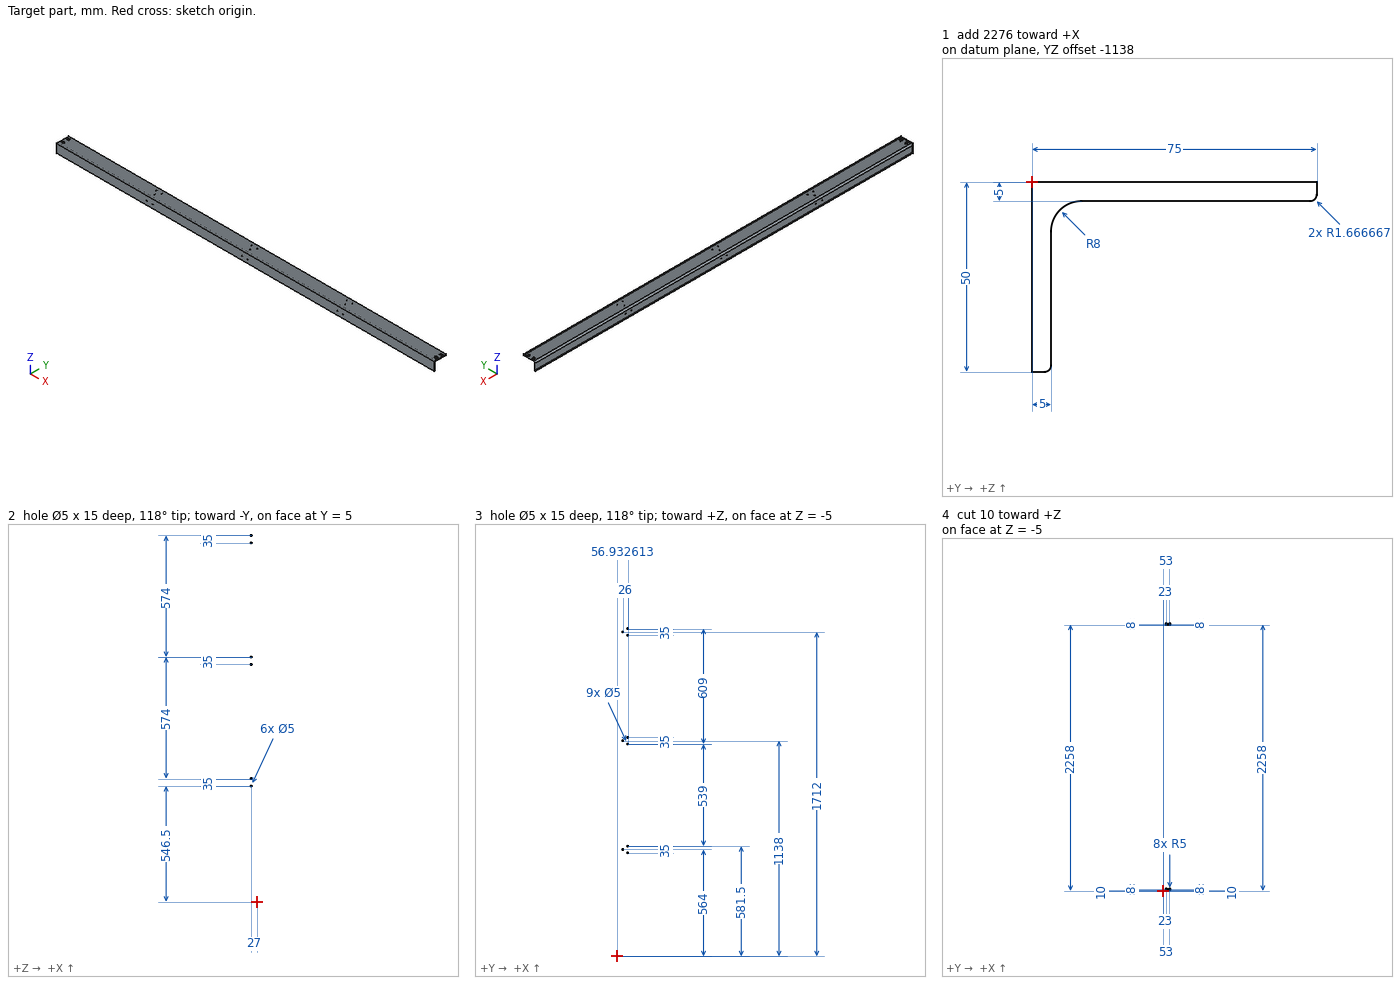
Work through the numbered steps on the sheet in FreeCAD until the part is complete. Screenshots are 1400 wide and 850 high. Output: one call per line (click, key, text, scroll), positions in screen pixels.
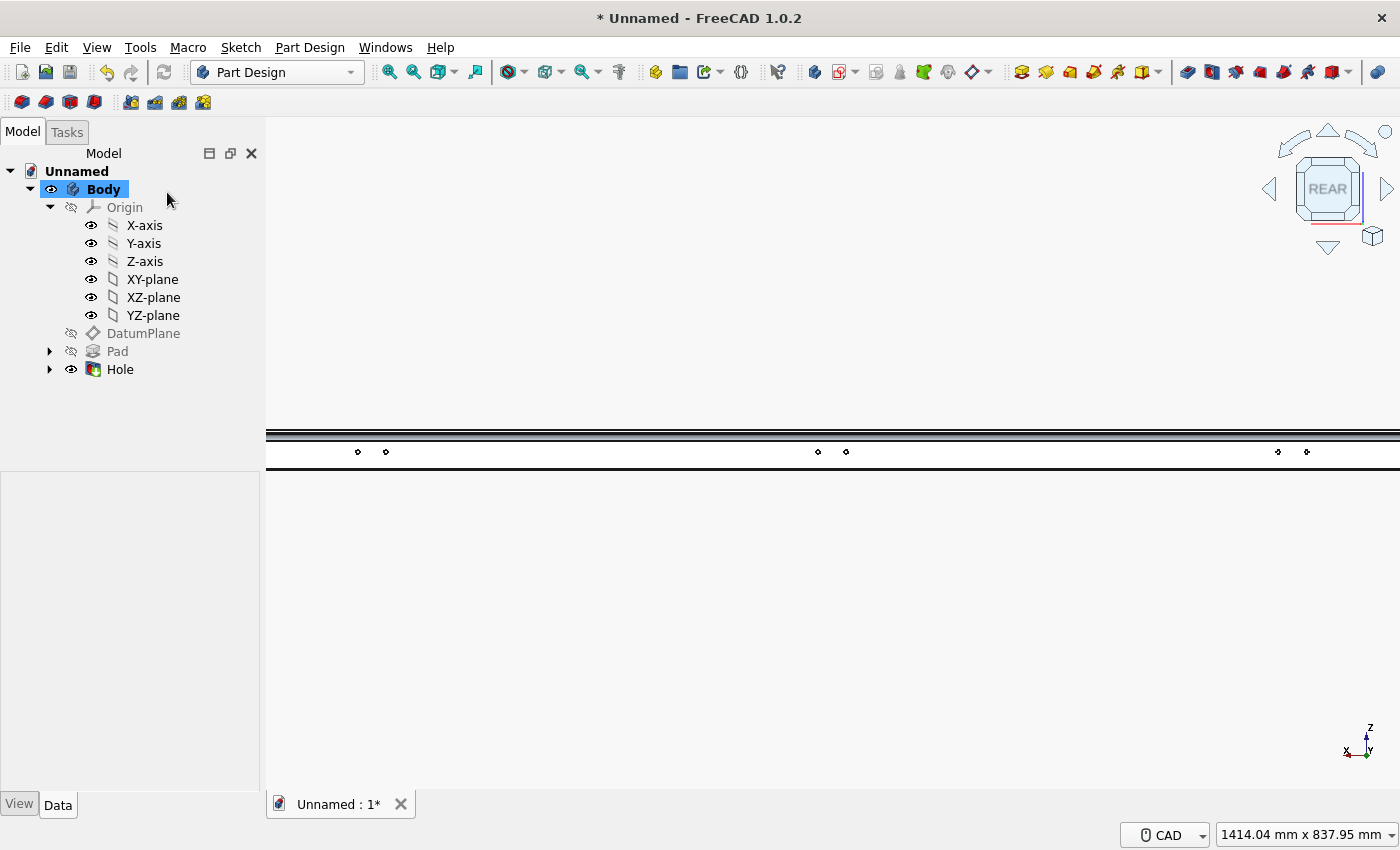
click(390, 72)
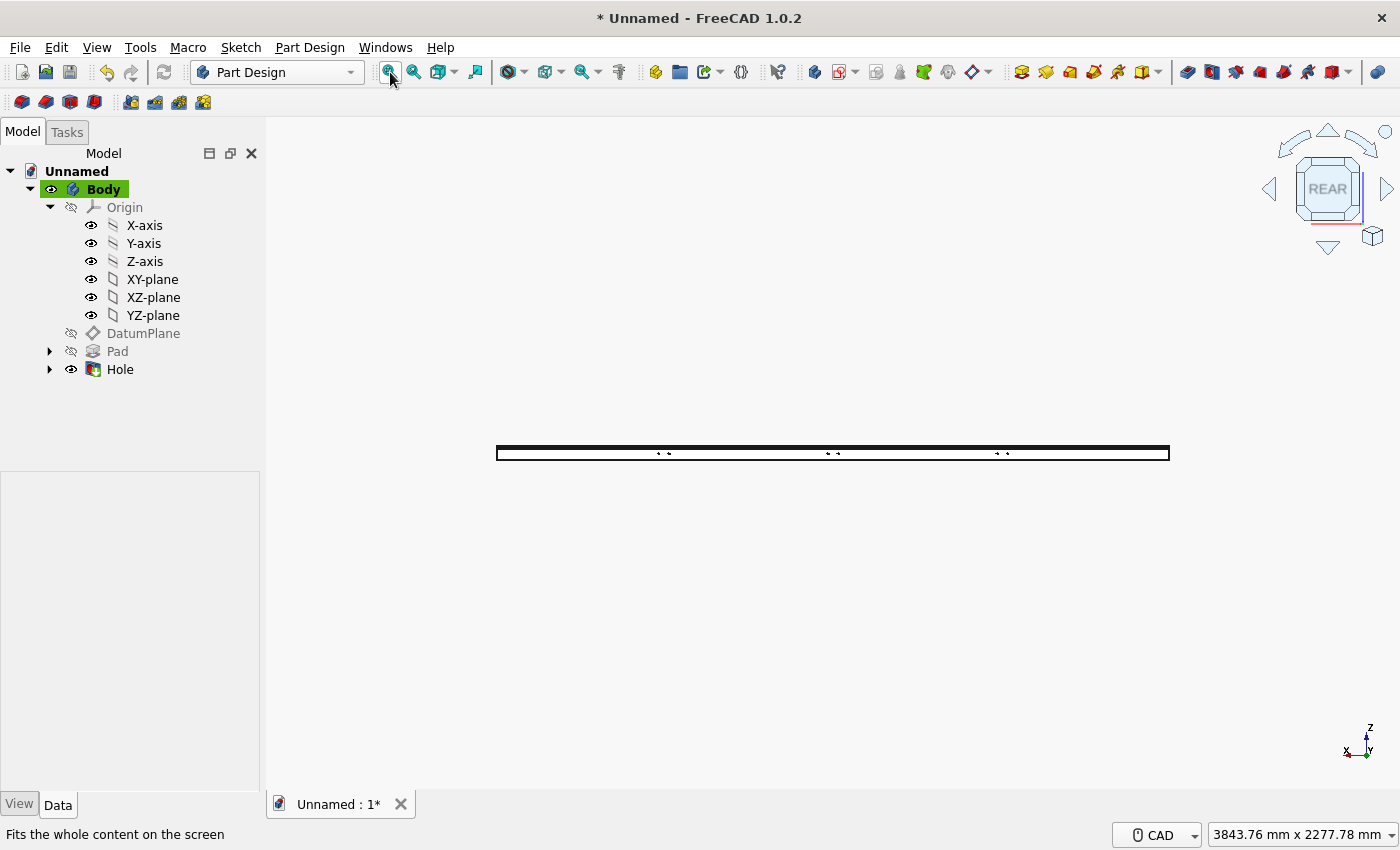
key(5)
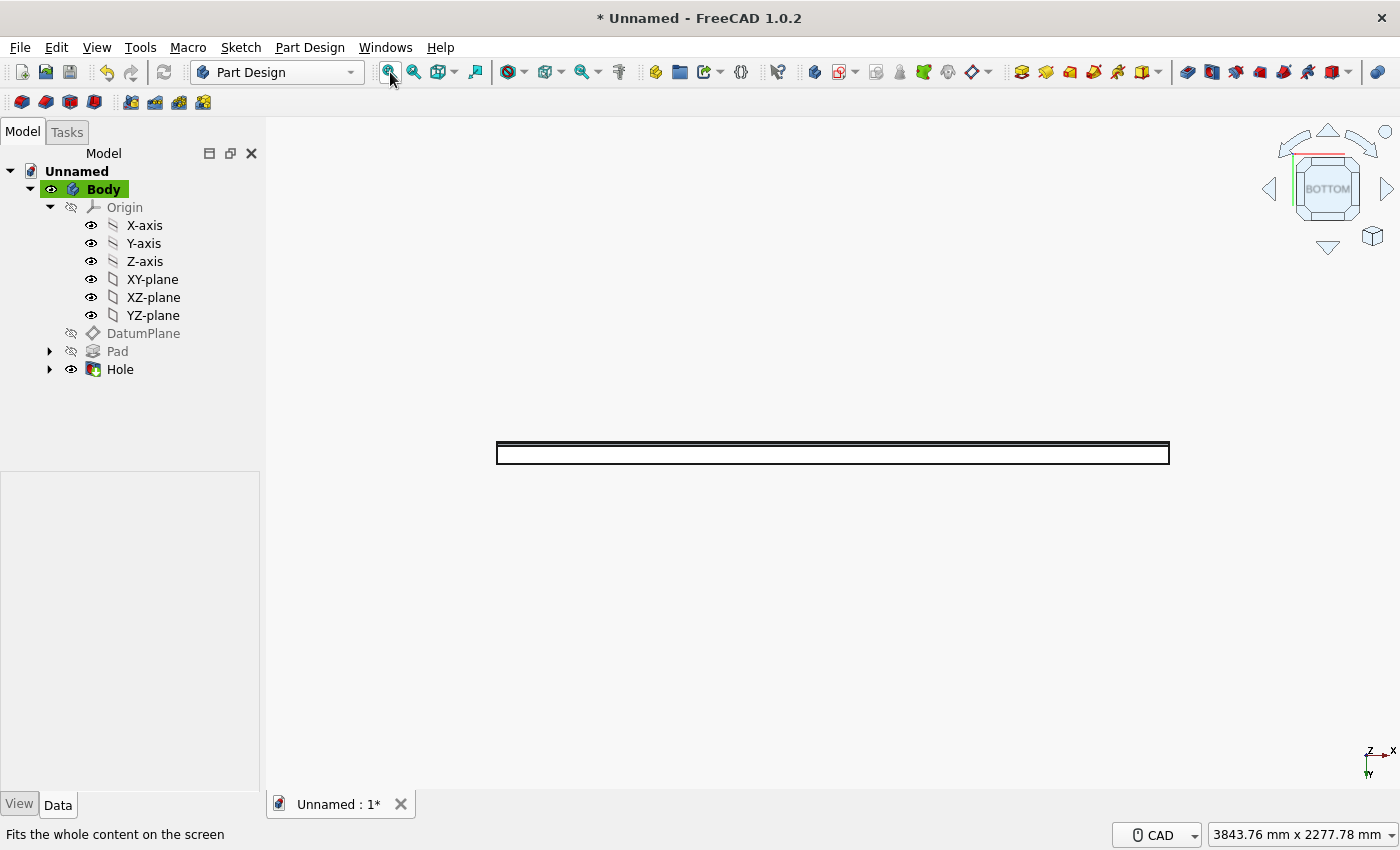
click(833, 454)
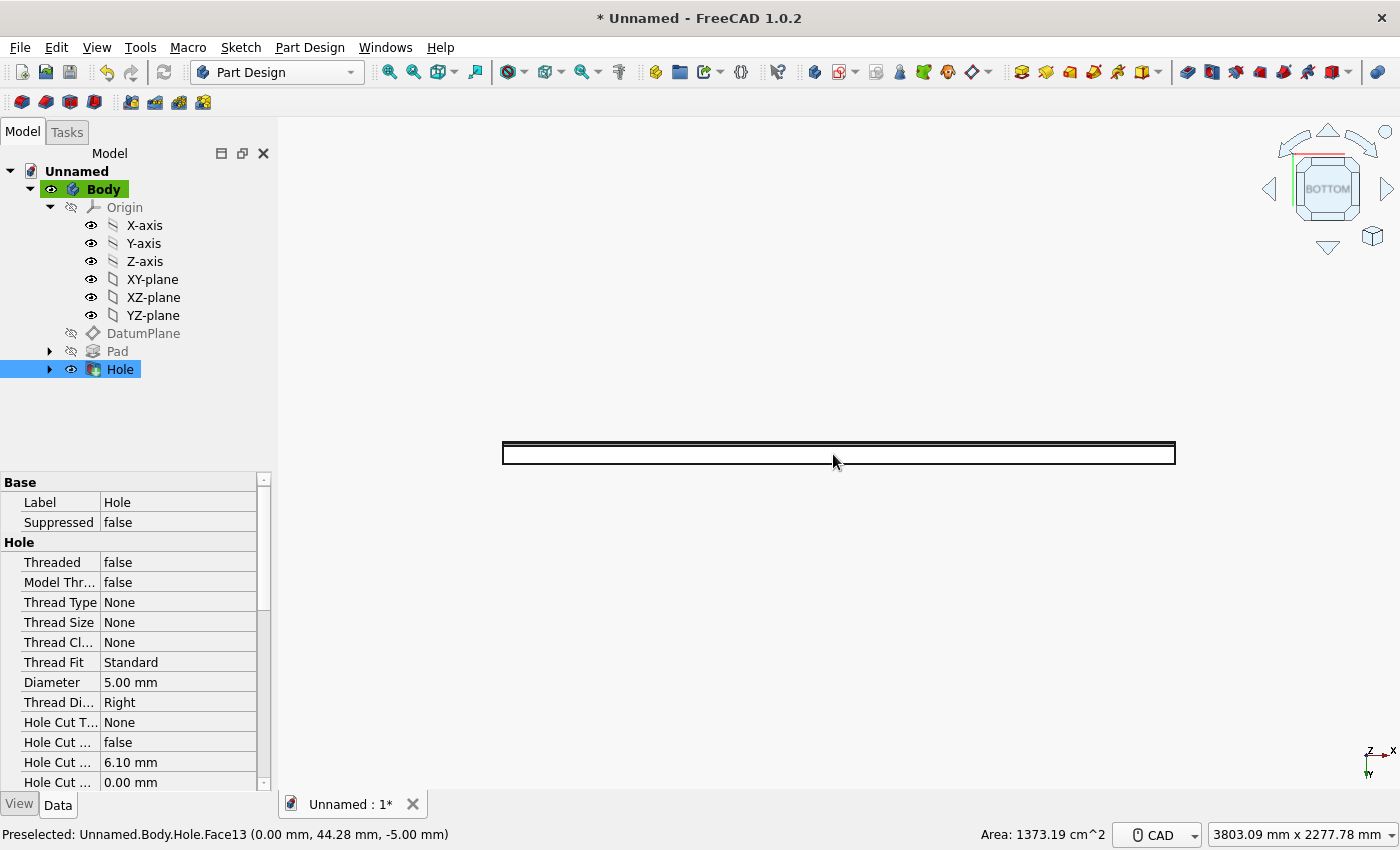
click(840, 72)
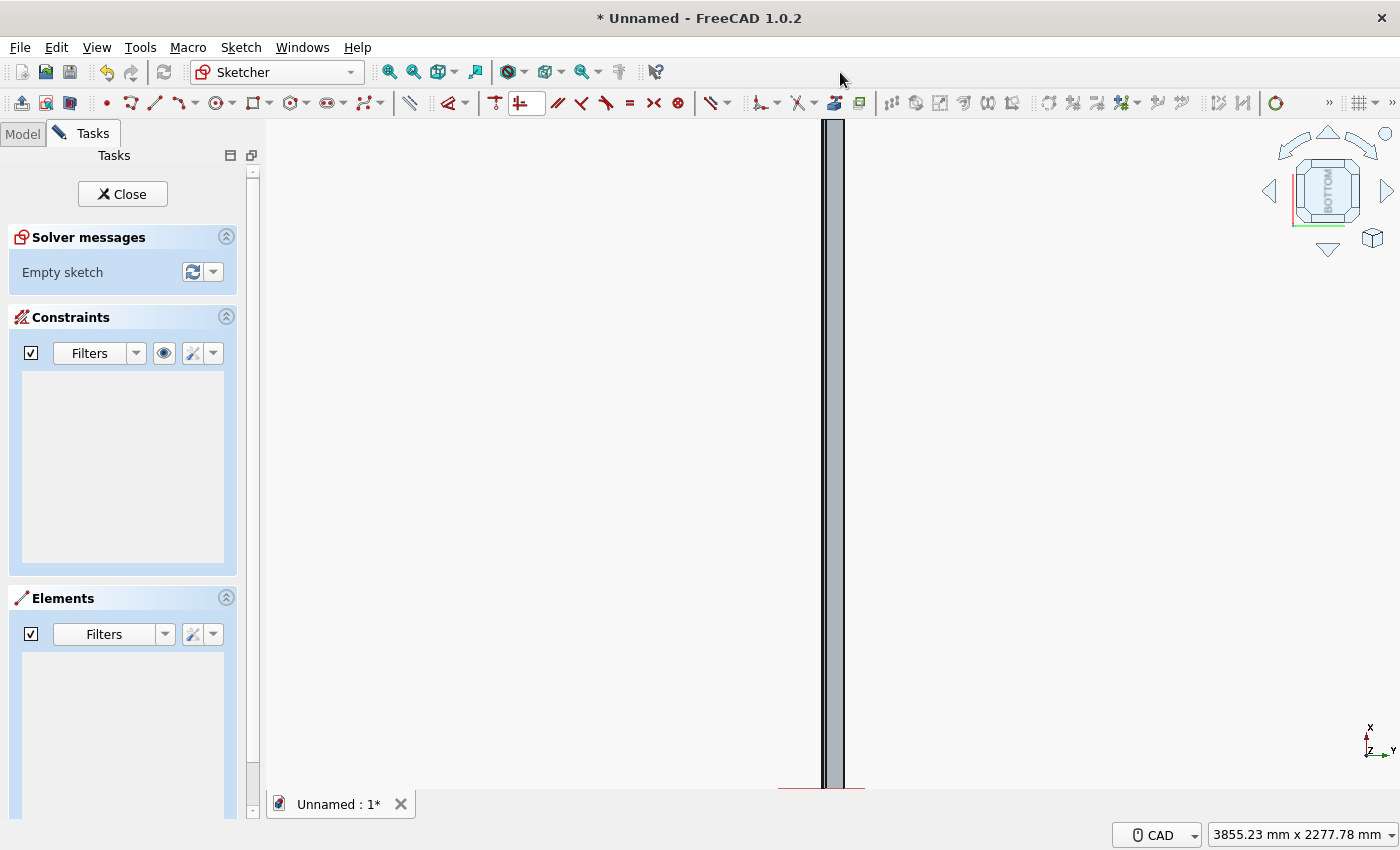
click(70, 104)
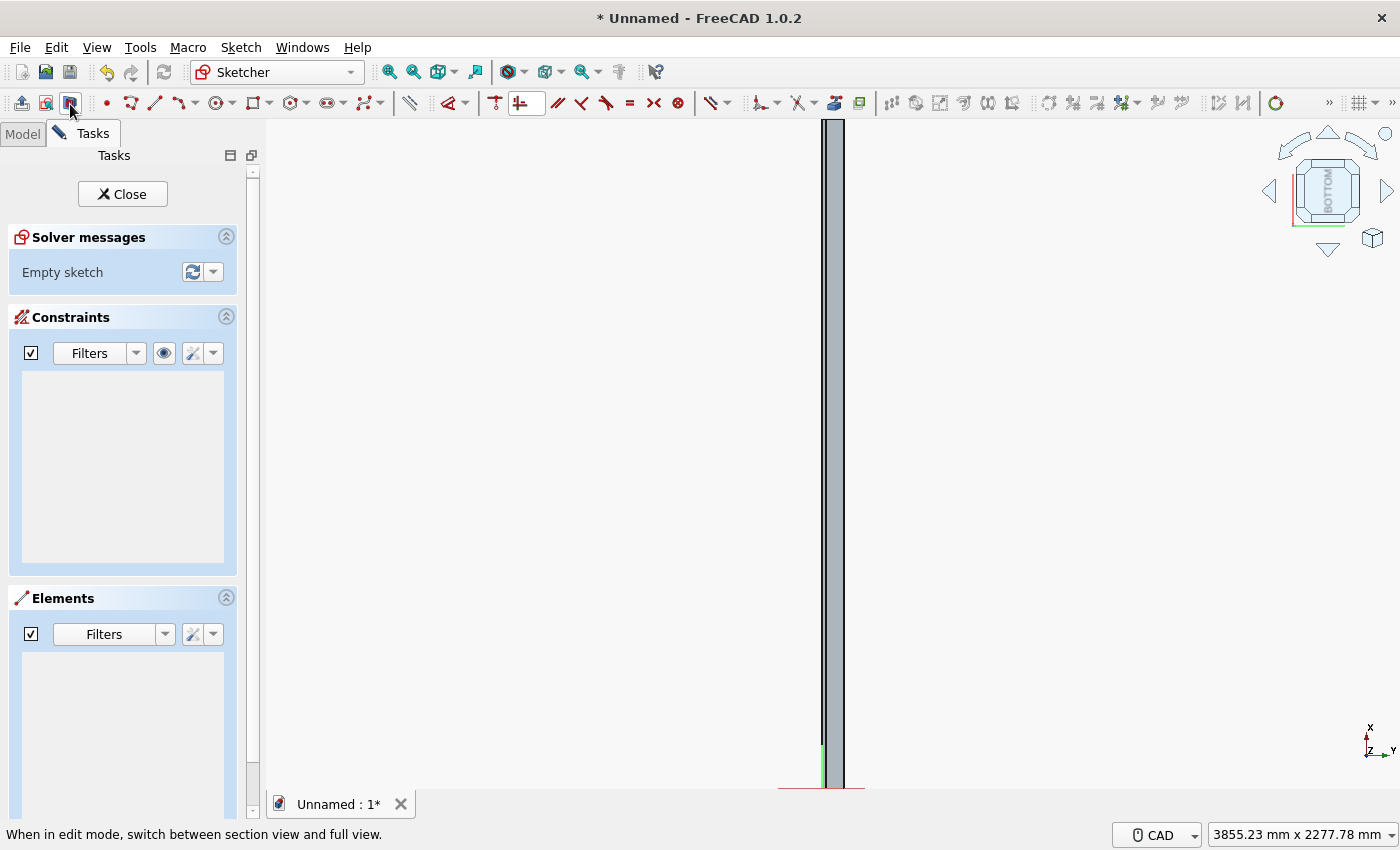
scroll(465, 147, down, 1)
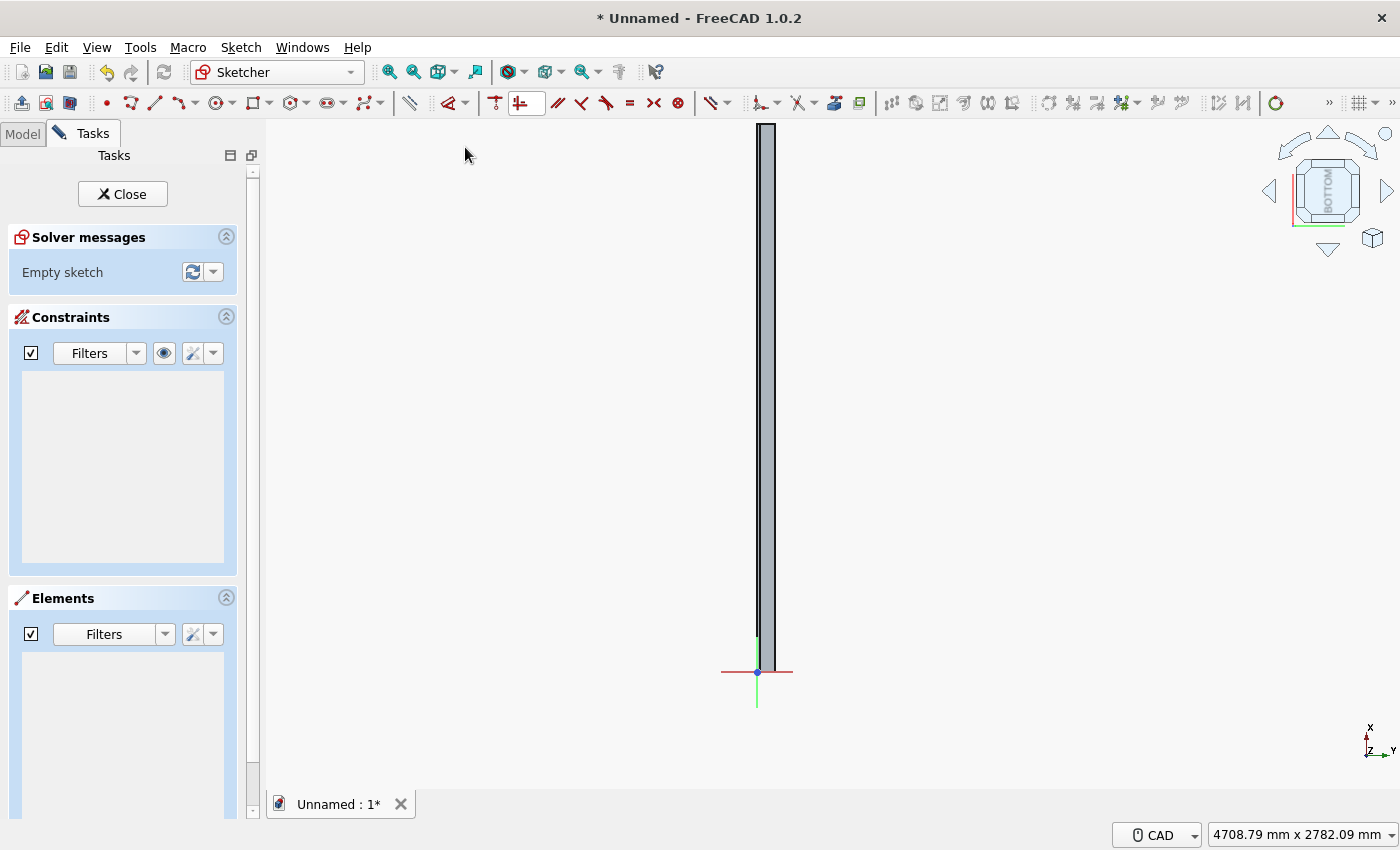
click(216, 104)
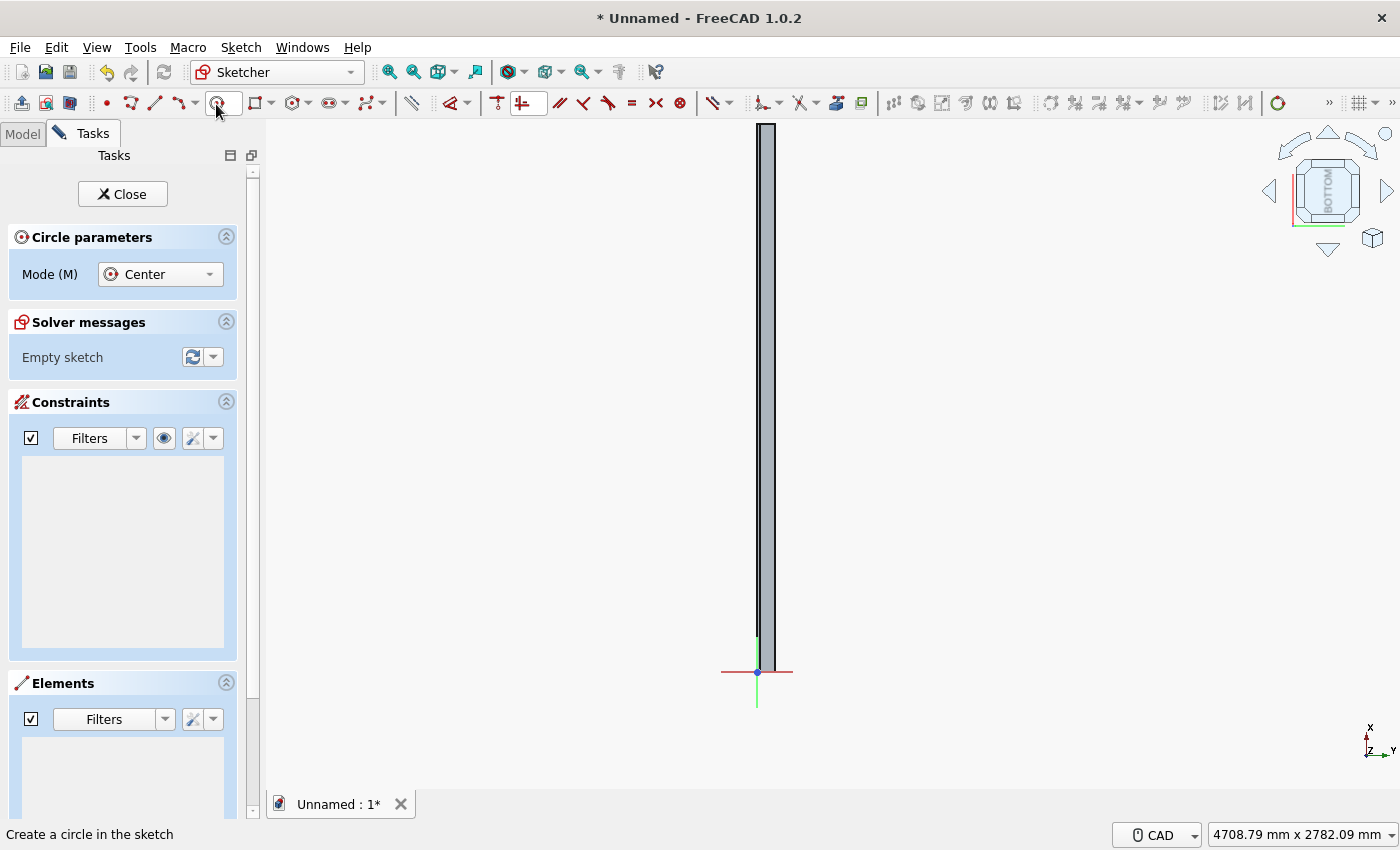
scroll(771, 403, up, 19)